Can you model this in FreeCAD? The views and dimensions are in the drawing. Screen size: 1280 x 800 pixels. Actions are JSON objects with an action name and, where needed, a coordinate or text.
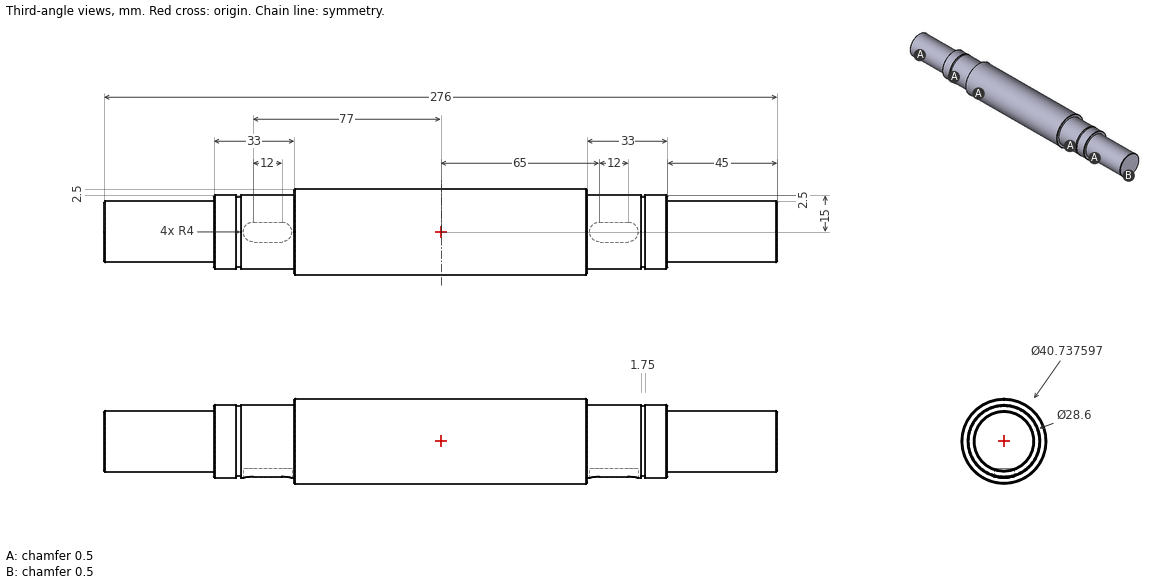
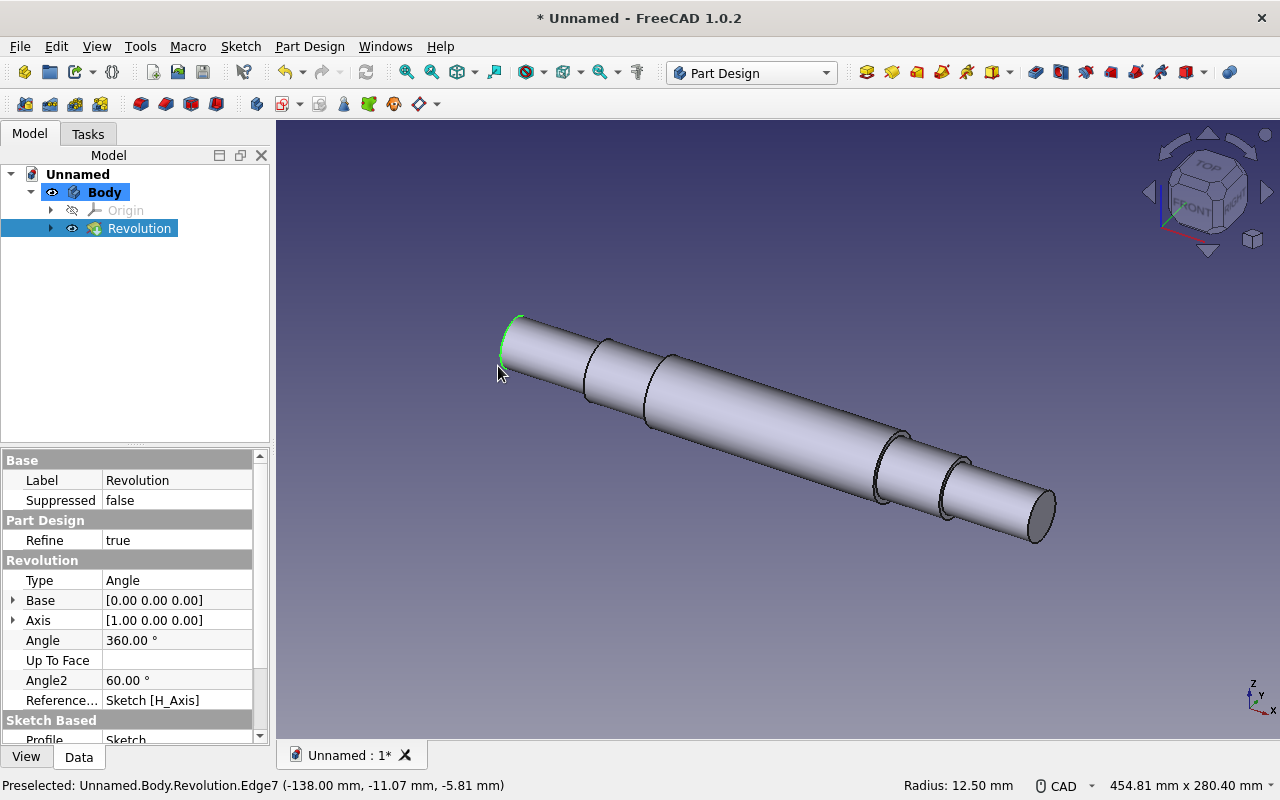
{"action": "left_click", "coordinate": [587, 399], "text": "ctrl"}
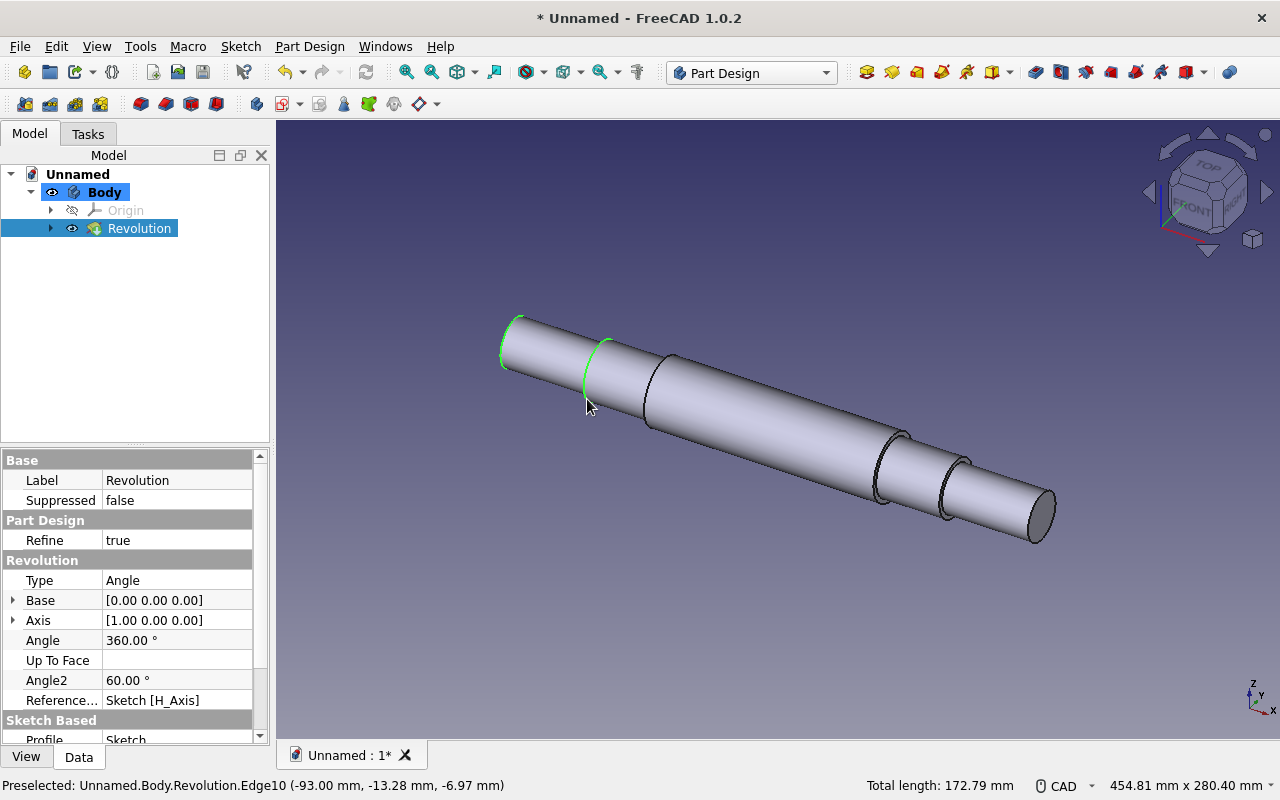
{"action": "left_click", "coordinate": [657, 366], "text": "ctrl"}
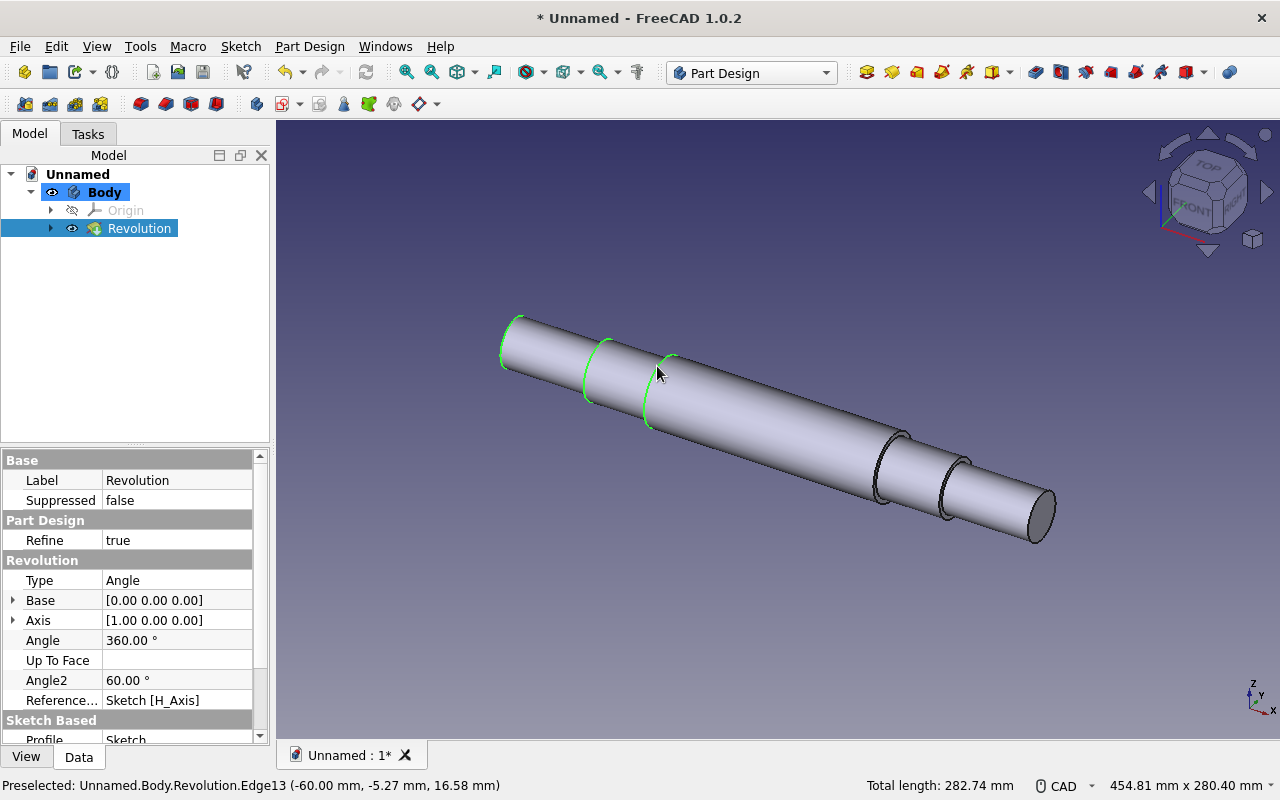
{"action": "left_click", "coordinate": [873, 486], "text": "ctrl"}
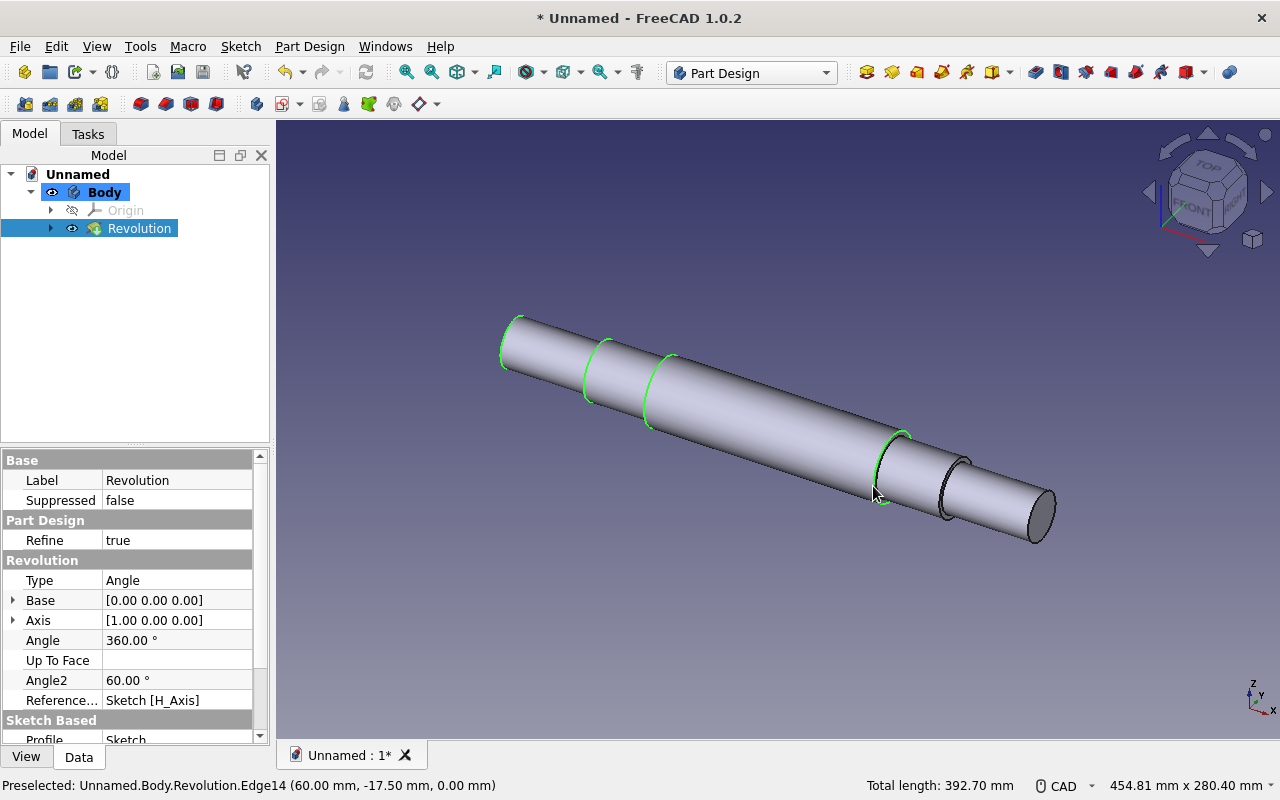
{"action": "left_click", "coordinate": [939, 504], "text": "ctrl"}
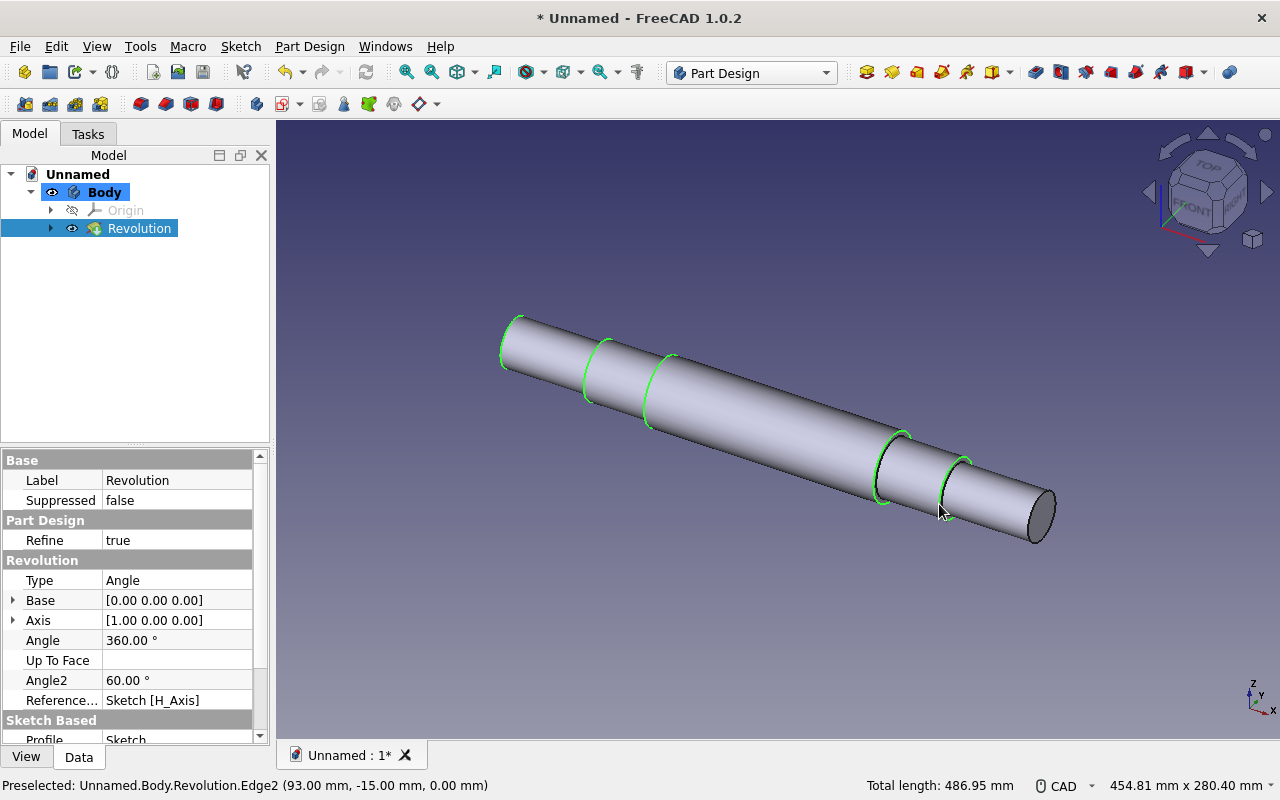
{"action": "left_click", "coordinate": [166, 104]}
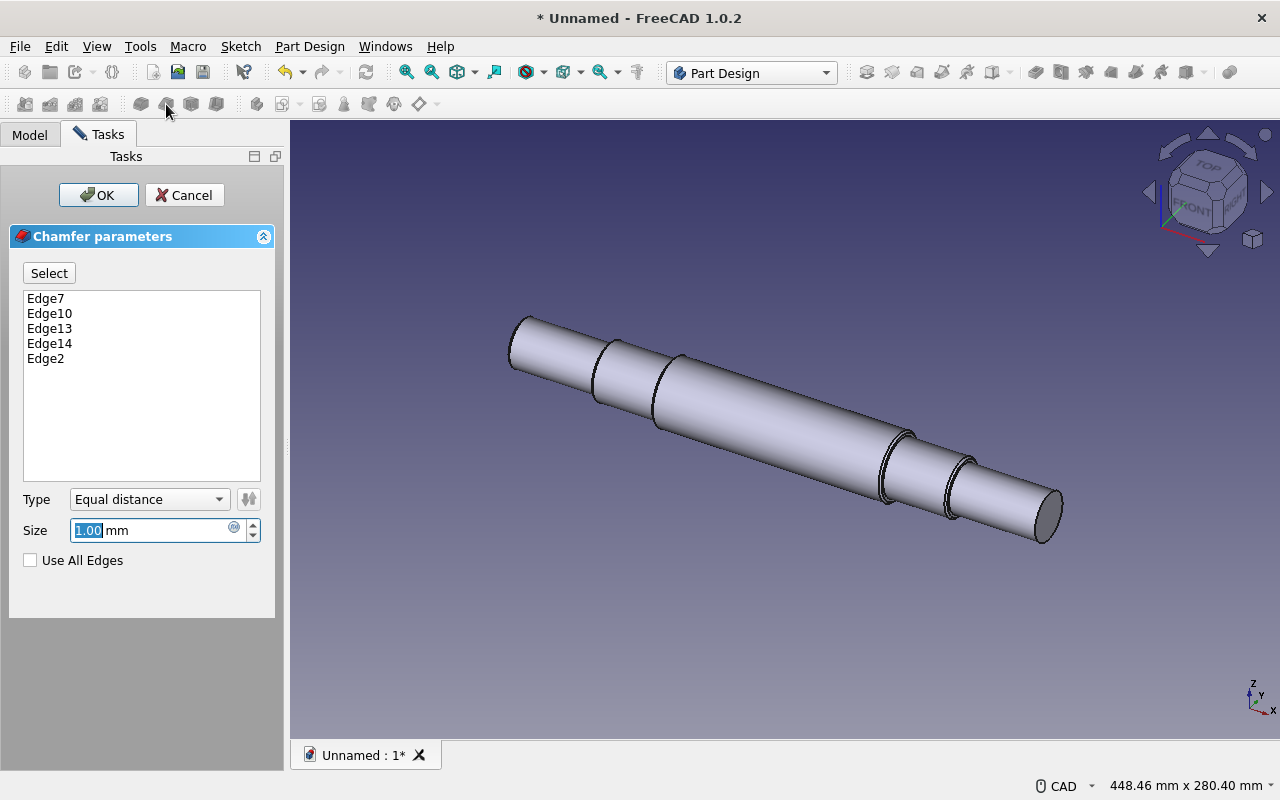
{"action": "type", "text": "0.5"}
{"action": "key", "text": "Tab"}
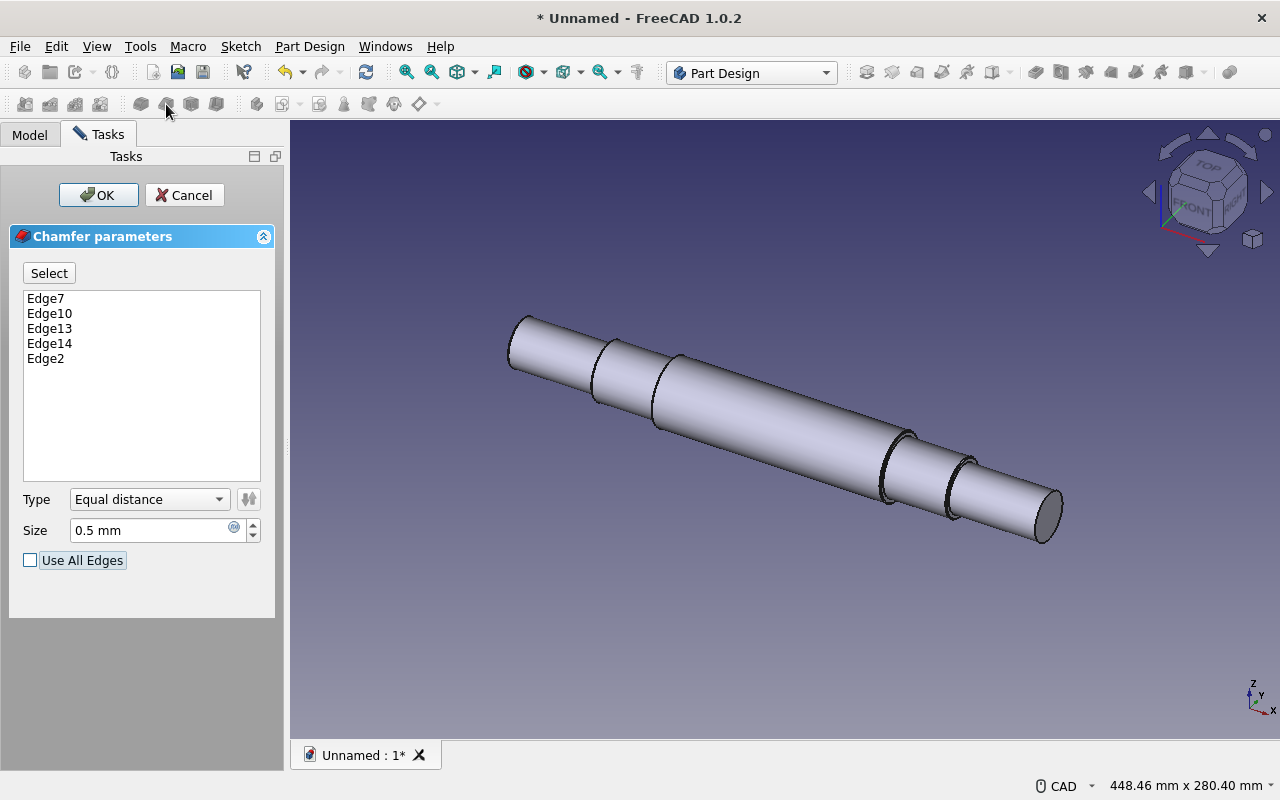
{"action": "left_click", "coordinate": [99, 195]}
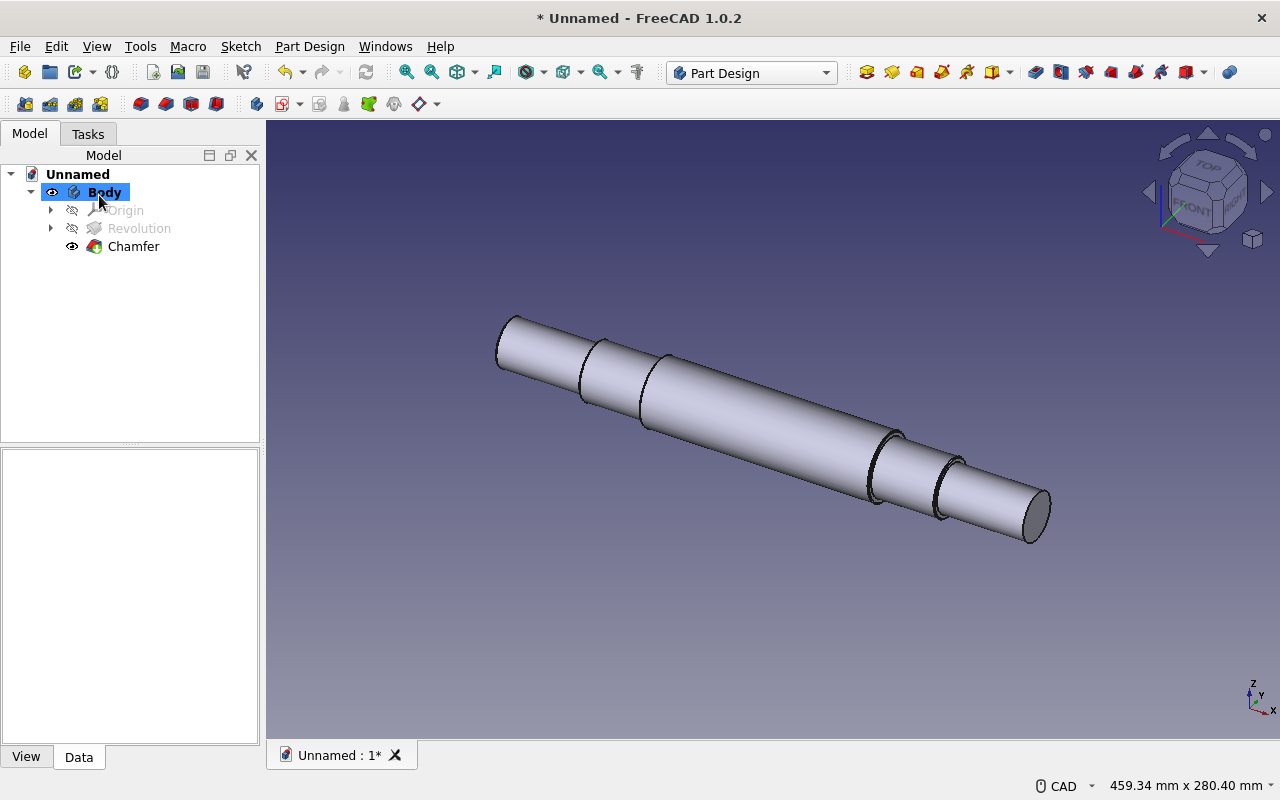
{"action": "left_click", "coordinate": [51, 210]}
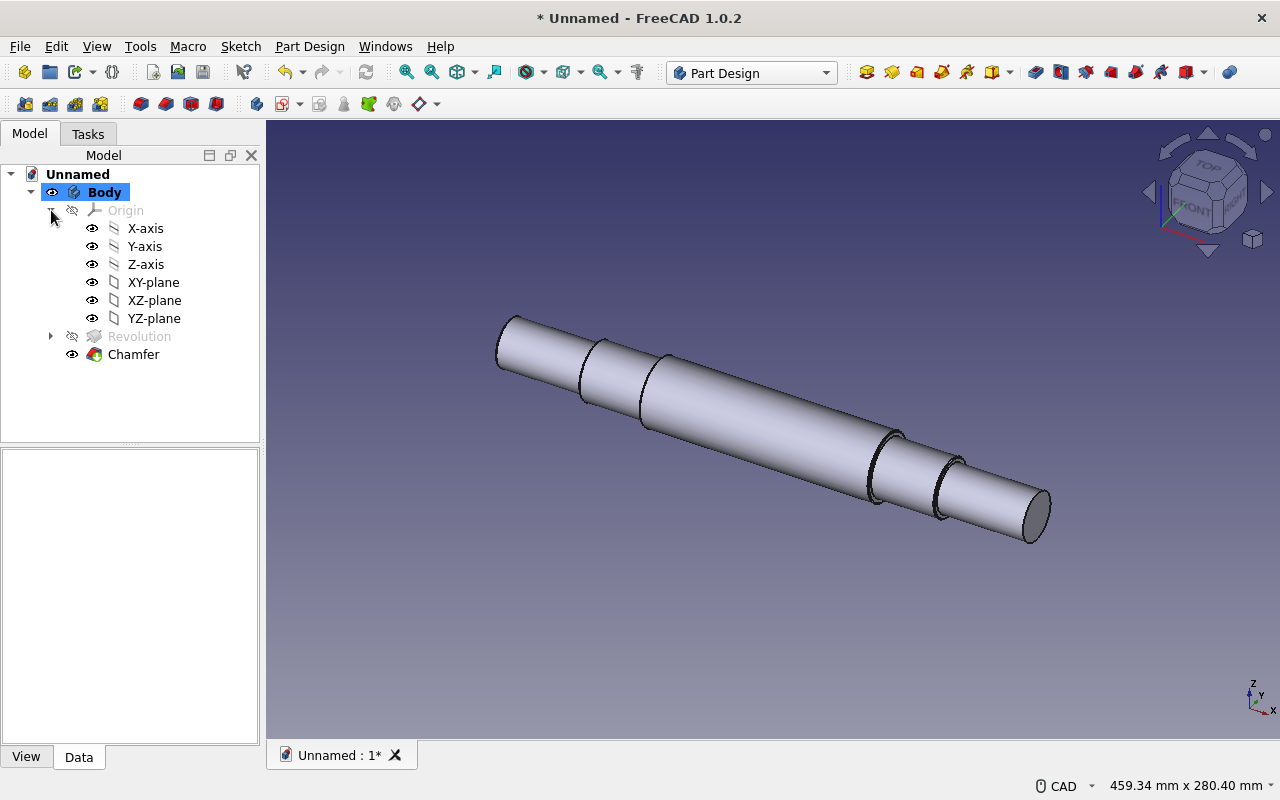
{"action": "left_click", "coordinate": [137, 282]}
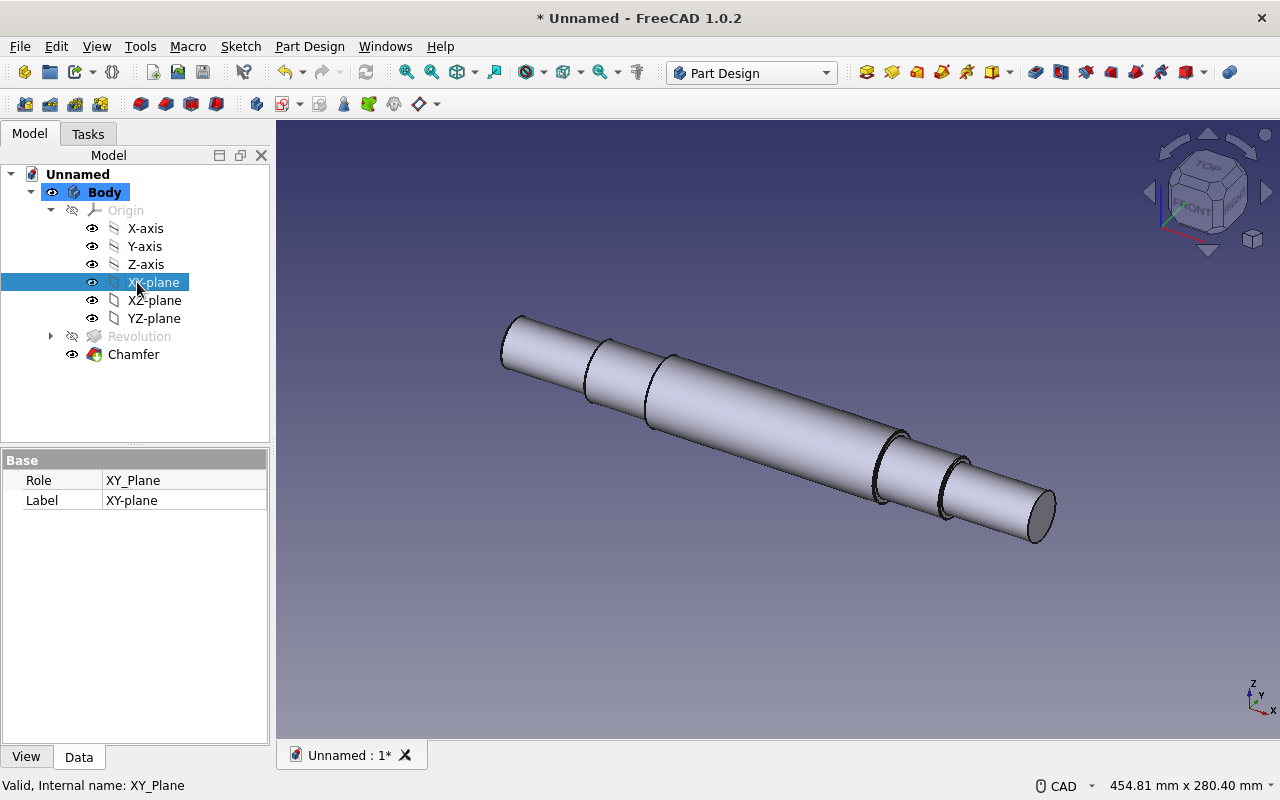
{"action": "left_click", "coordinate": [418, 104]}